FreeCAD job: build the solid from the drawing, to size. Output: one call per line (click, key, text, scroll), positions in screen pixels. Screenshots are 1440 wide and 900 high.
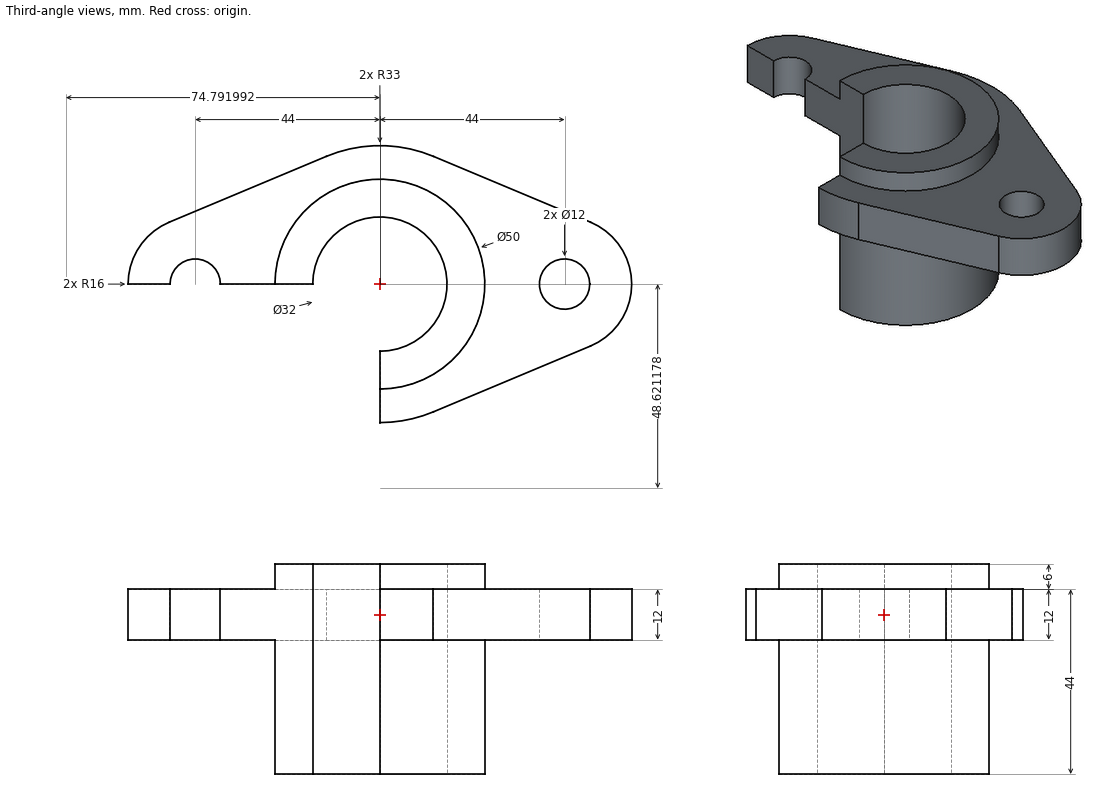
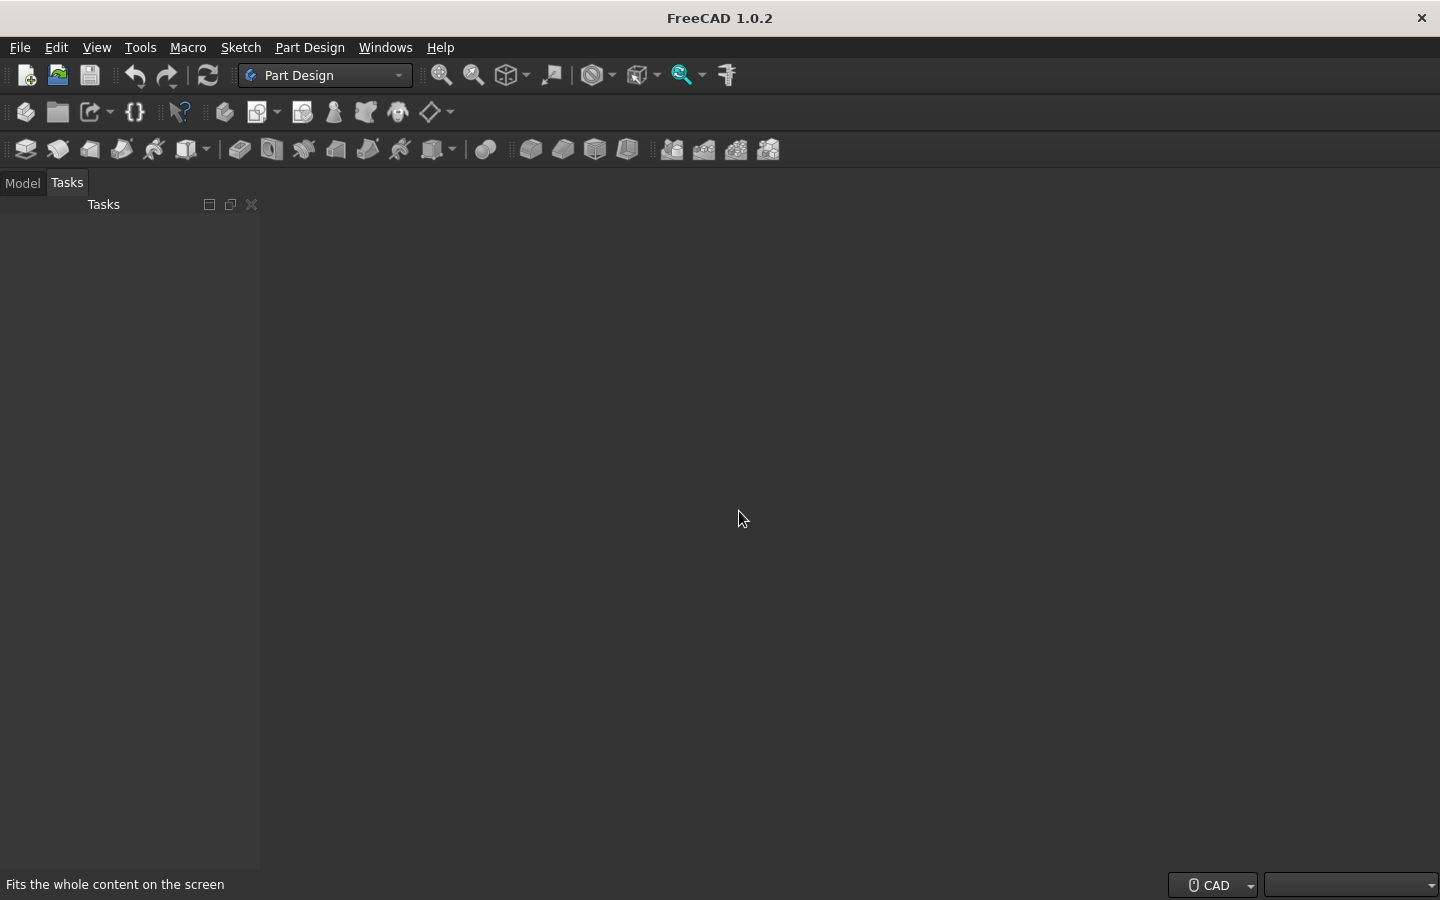
click(26, 76)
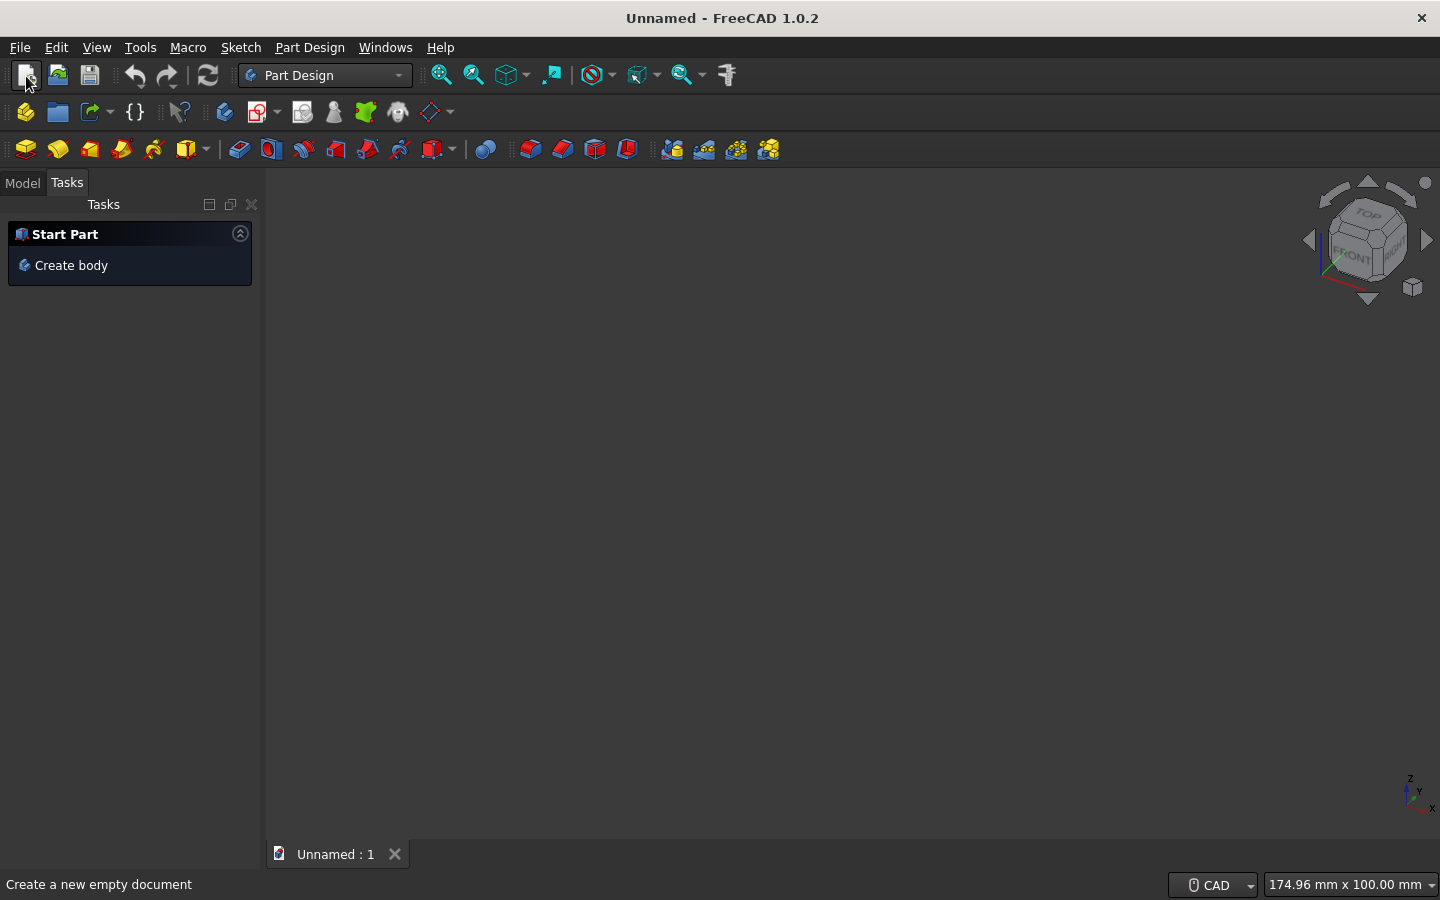
click(258, 112)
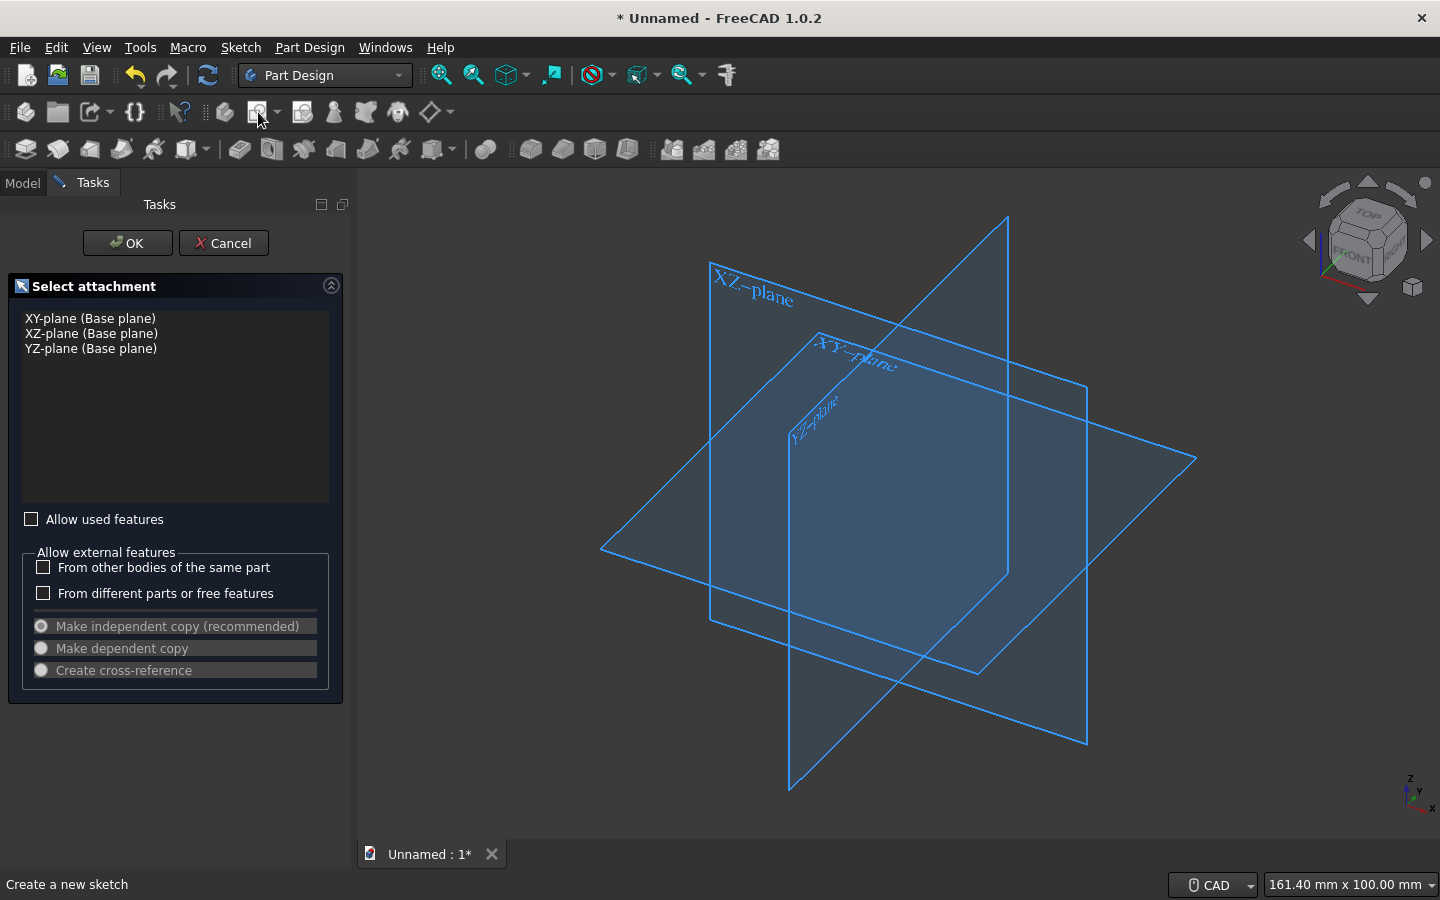
click(82, 318)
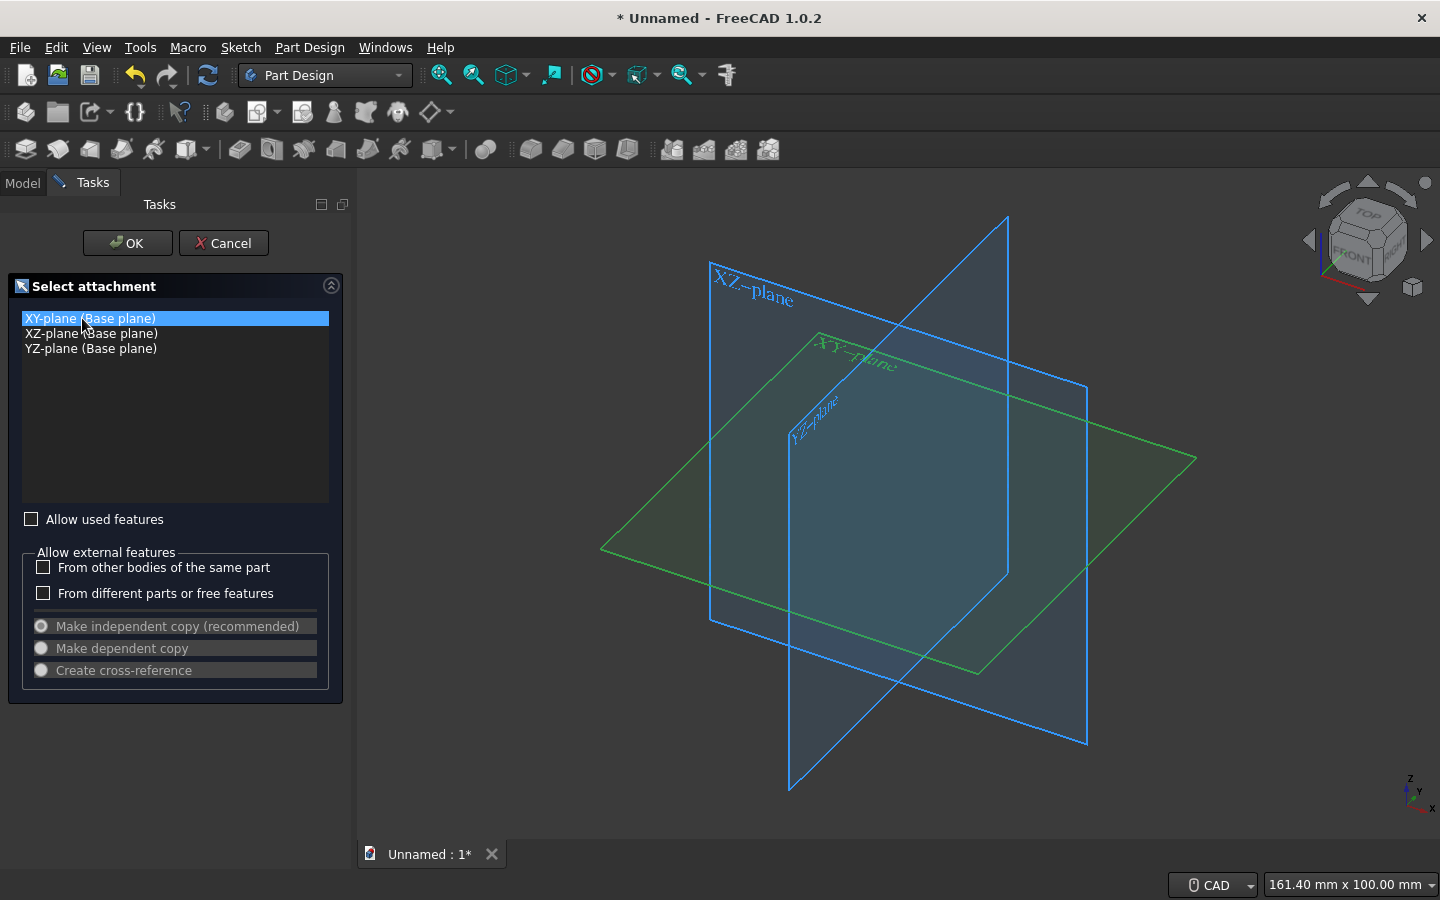
click(128, 243)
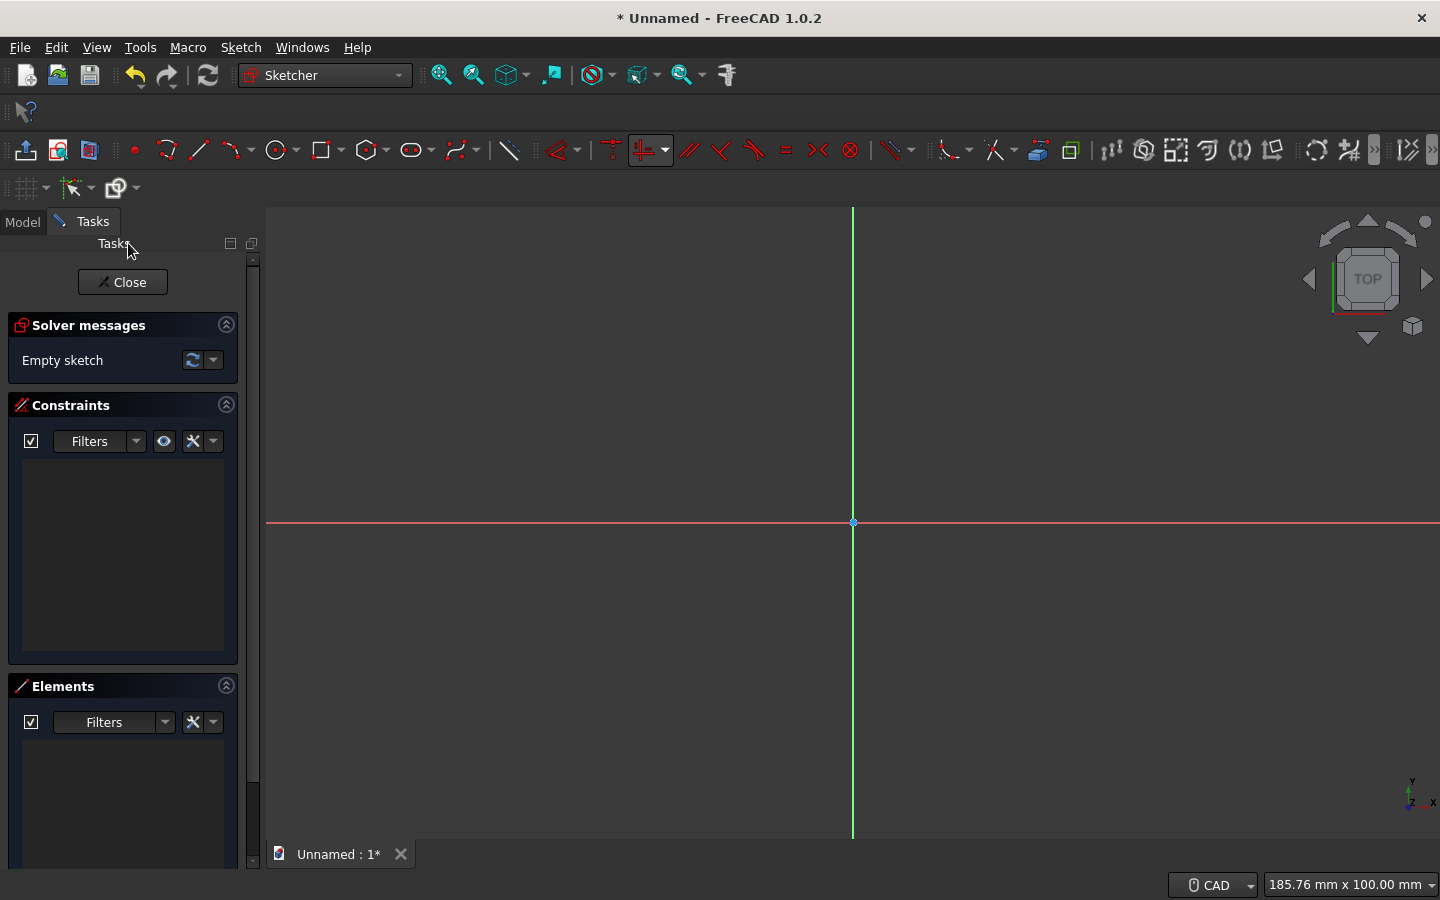
click(200, 150)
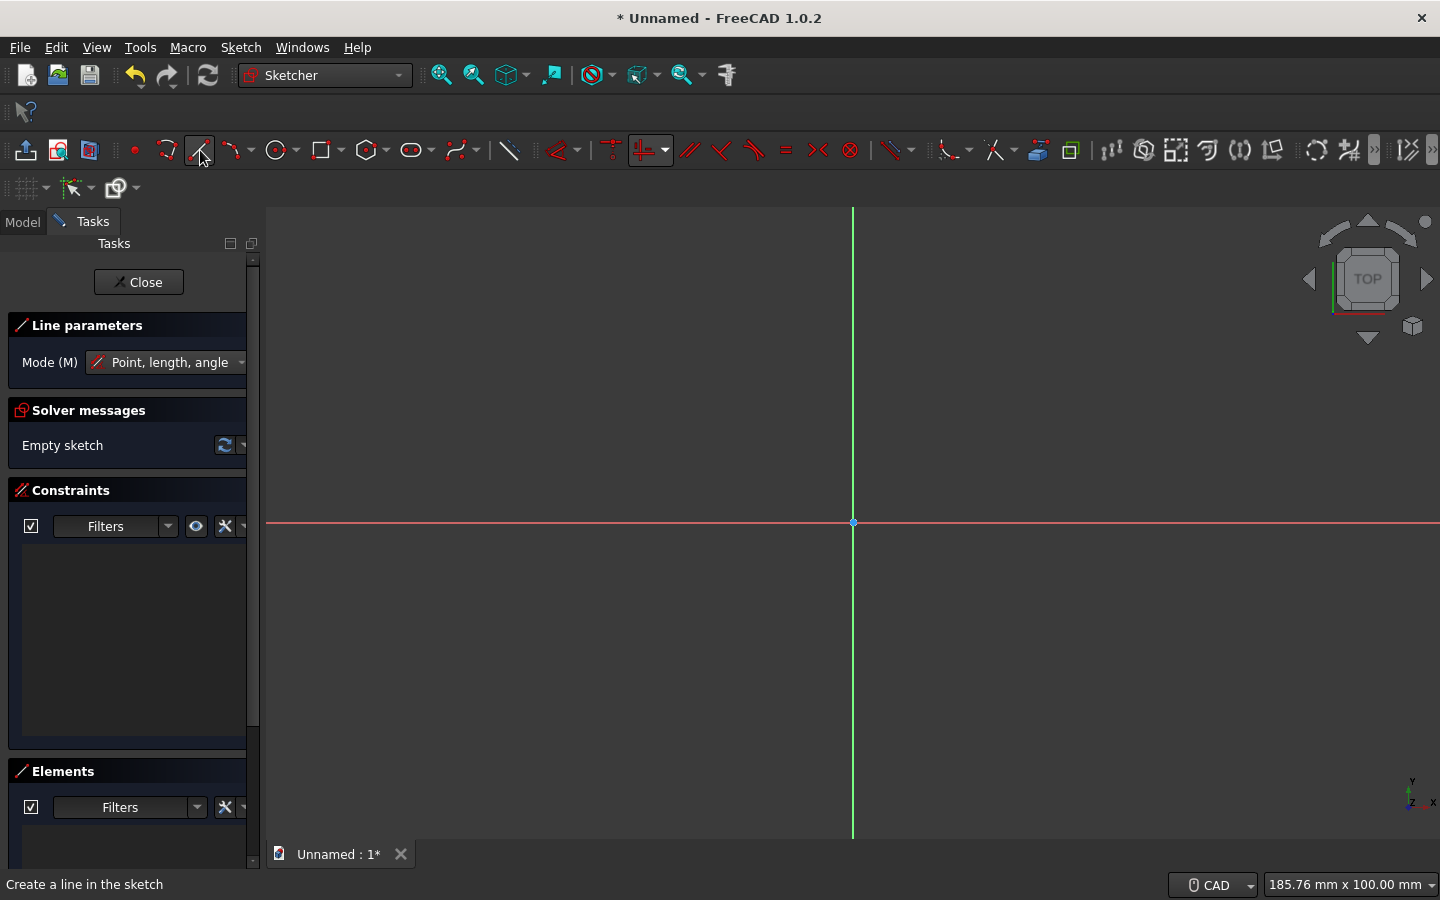
click(1170, 430)
click(934, 331)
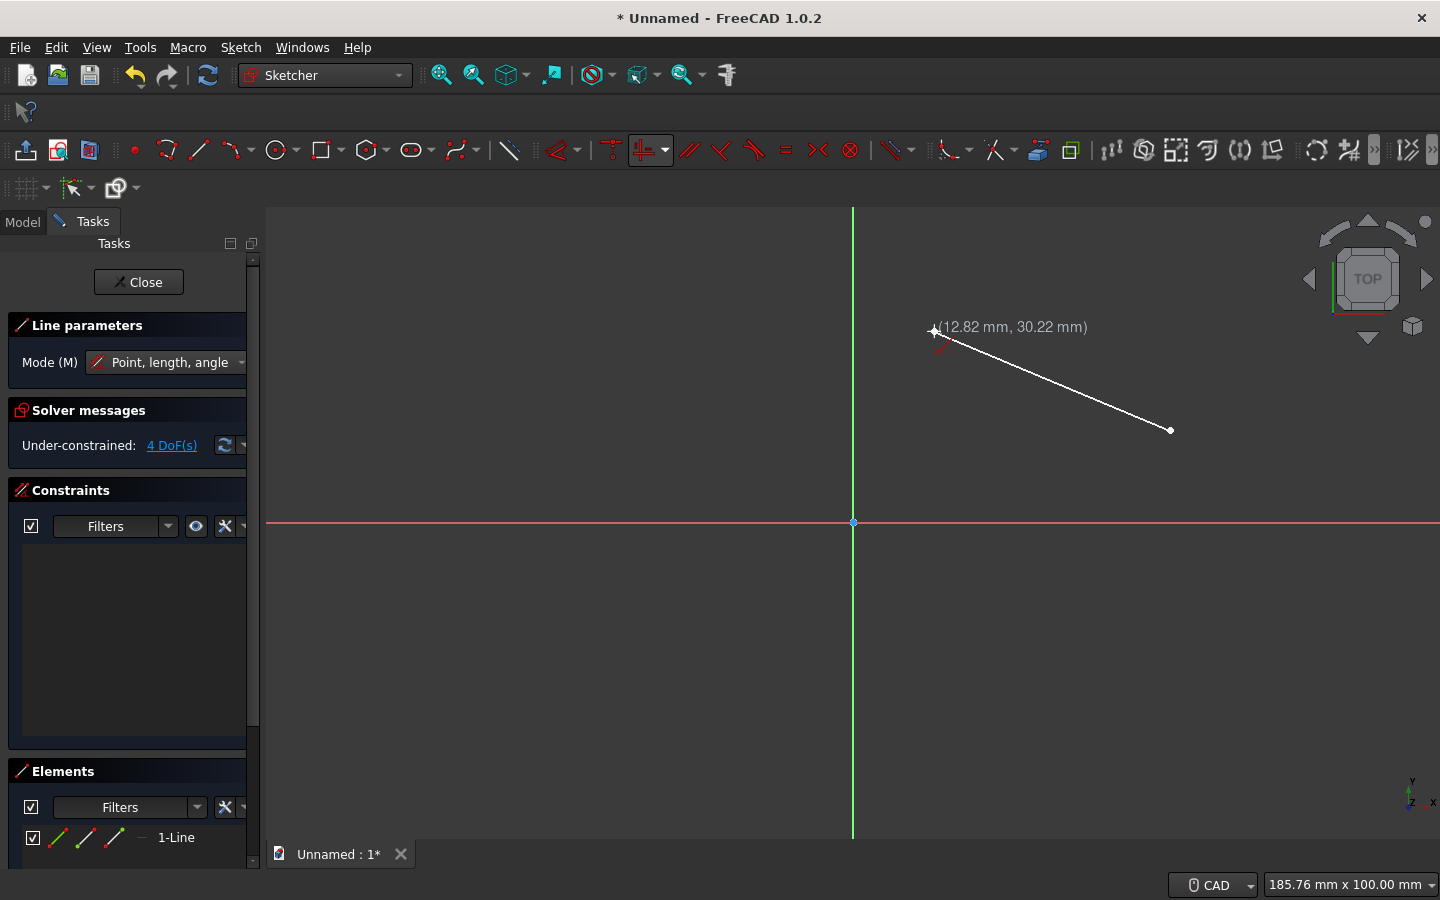
click(772, 331)
click(536, 430)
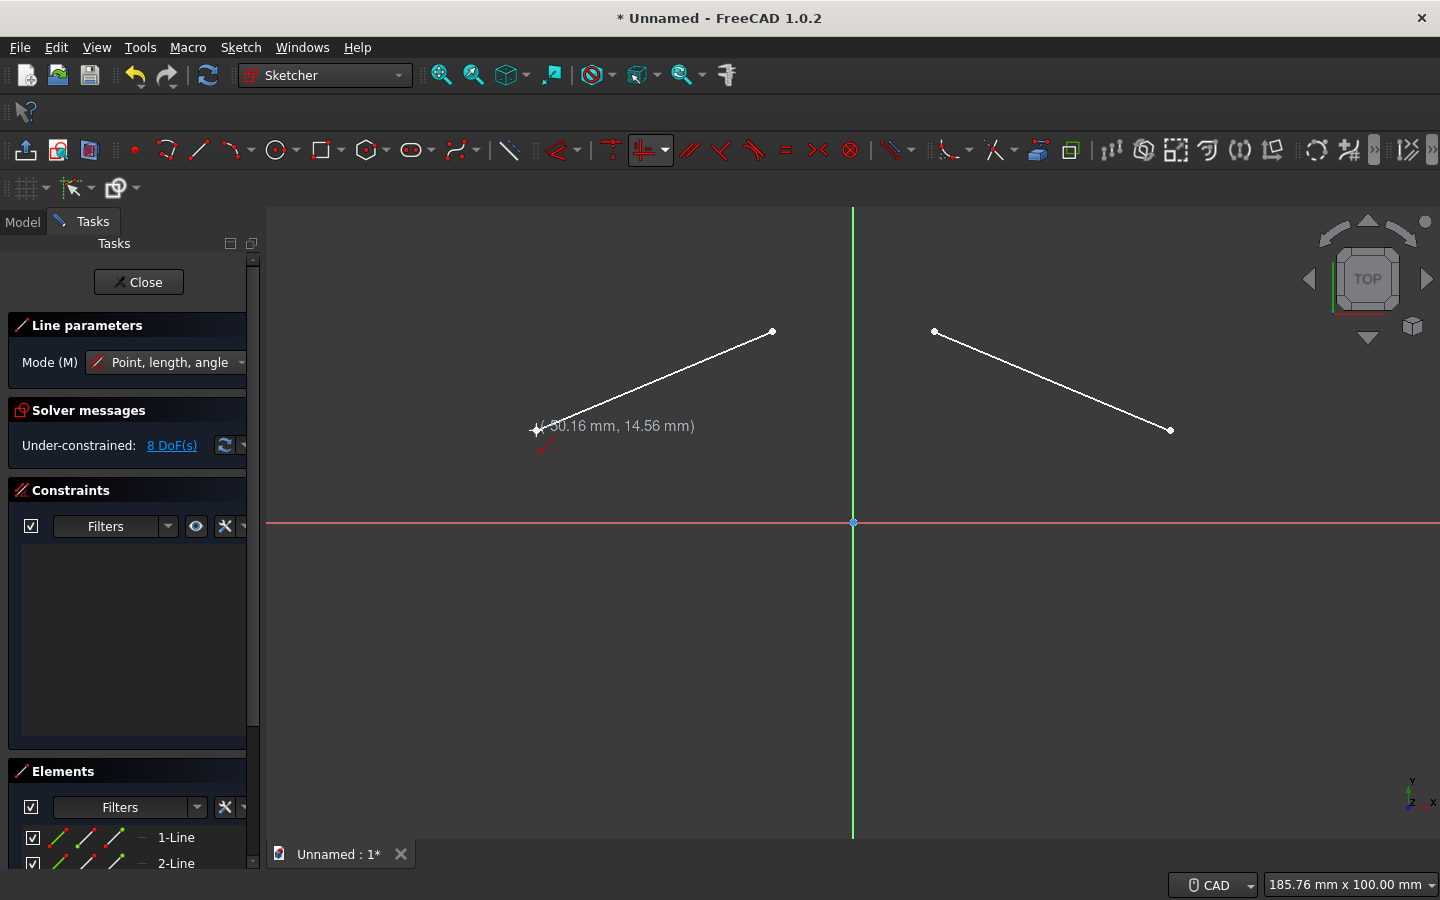
click(536, 616)
click(772, 715)